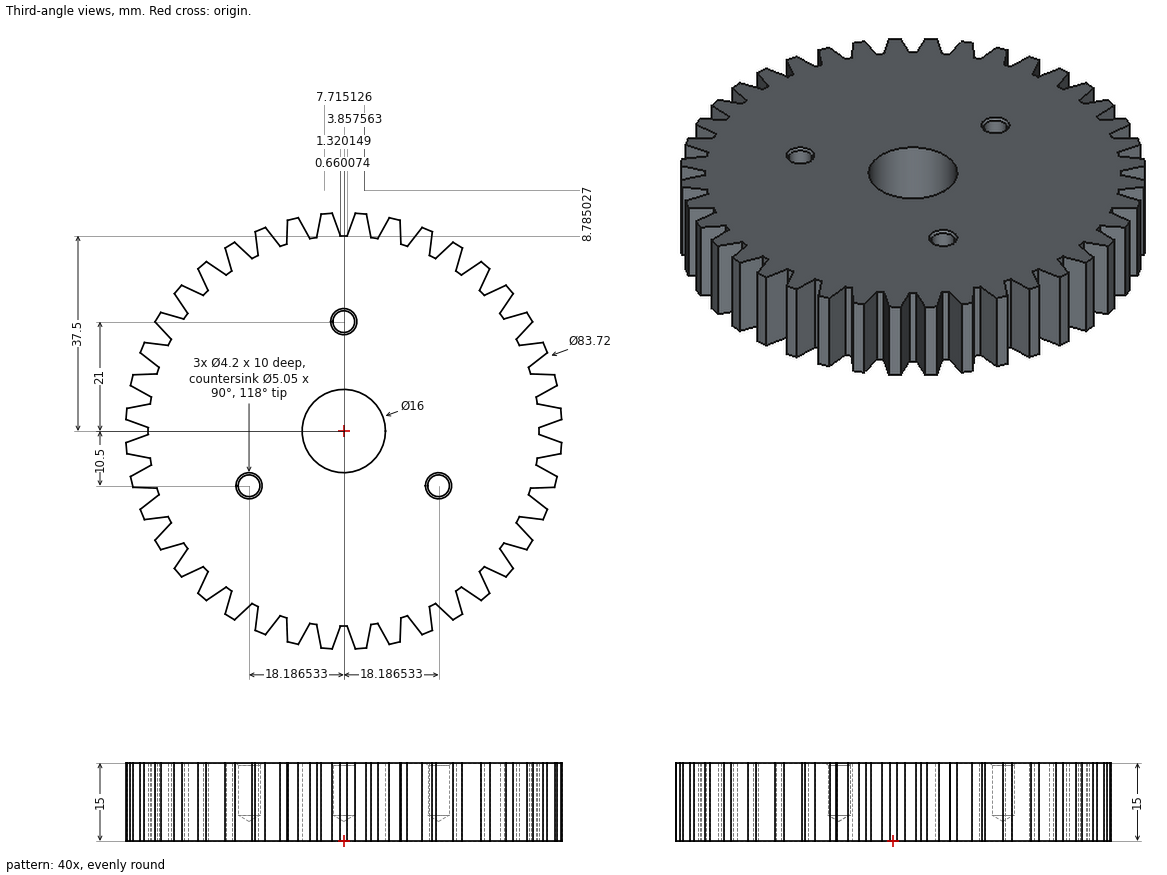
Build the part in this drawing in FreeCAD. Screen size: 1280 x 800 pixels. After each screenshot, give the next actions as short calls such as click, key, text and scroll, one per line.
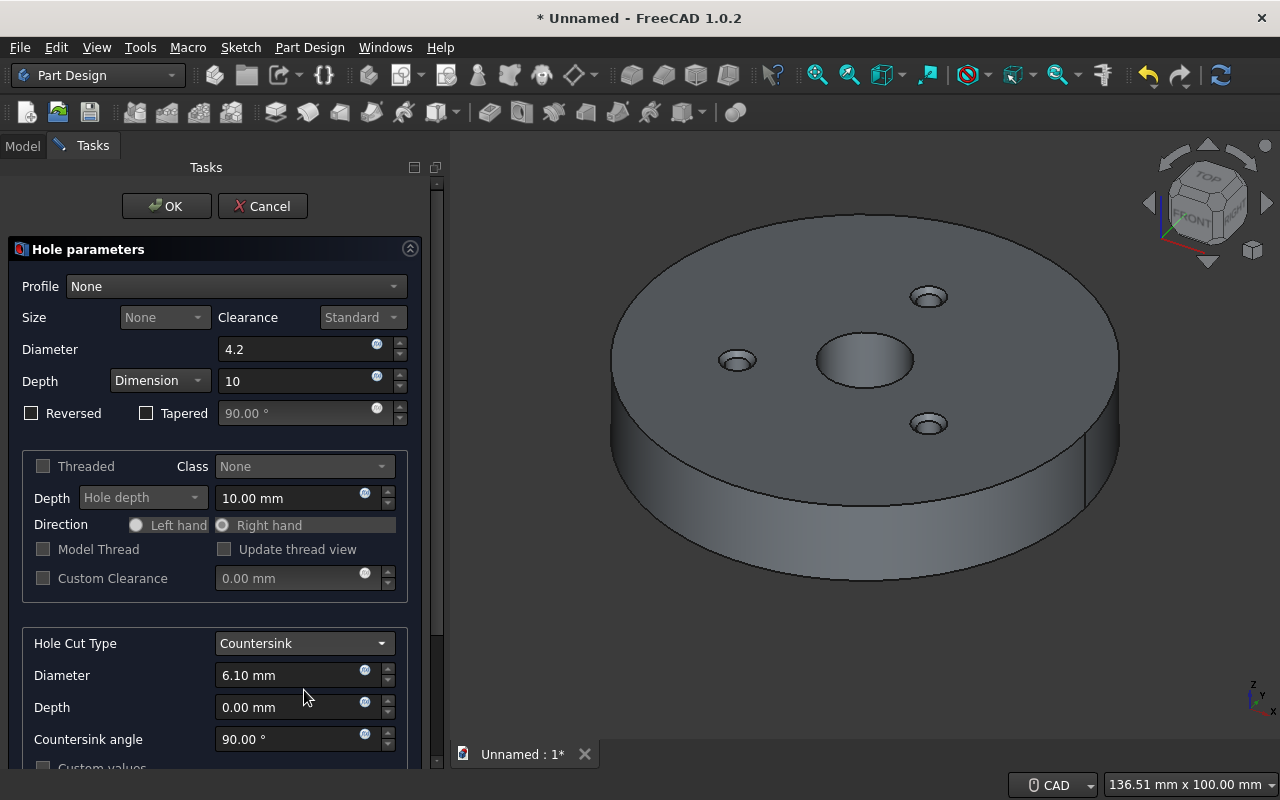
triple_click(298, 675)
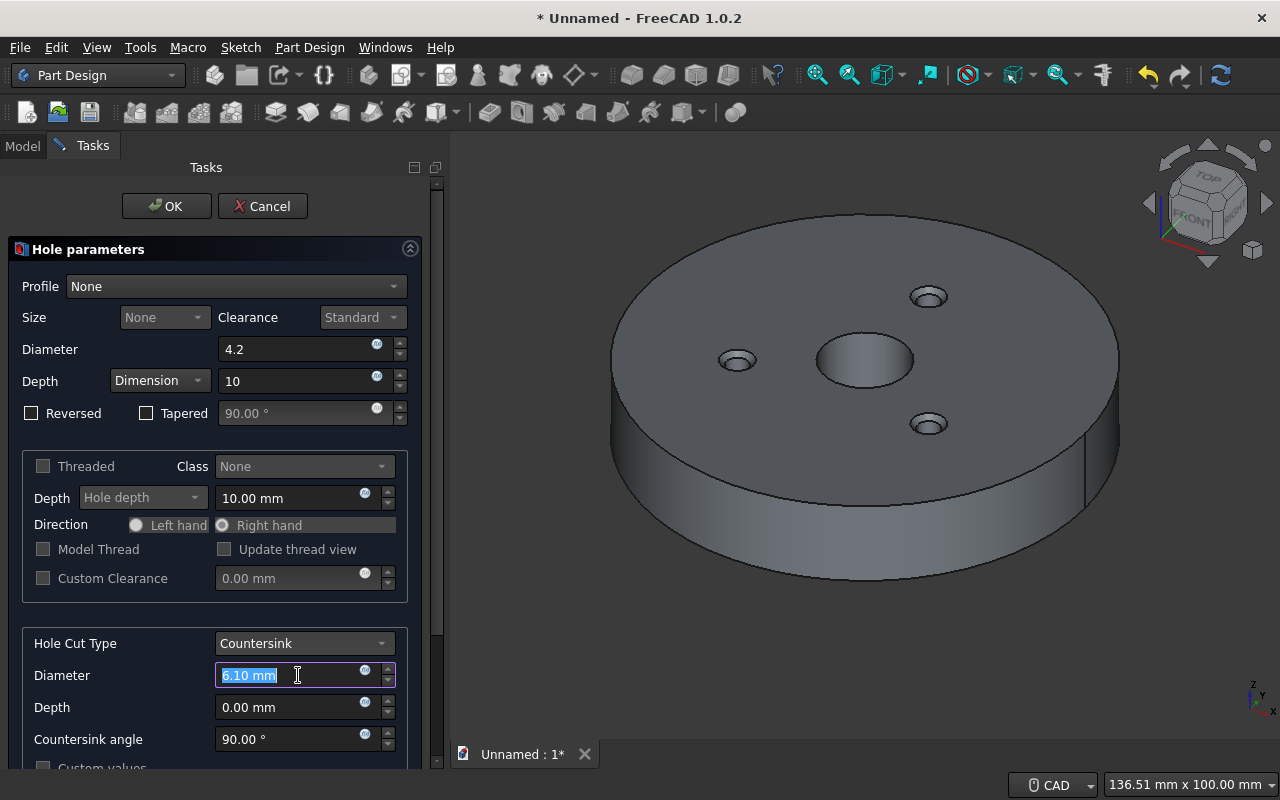
text(5.05)
key(Tab)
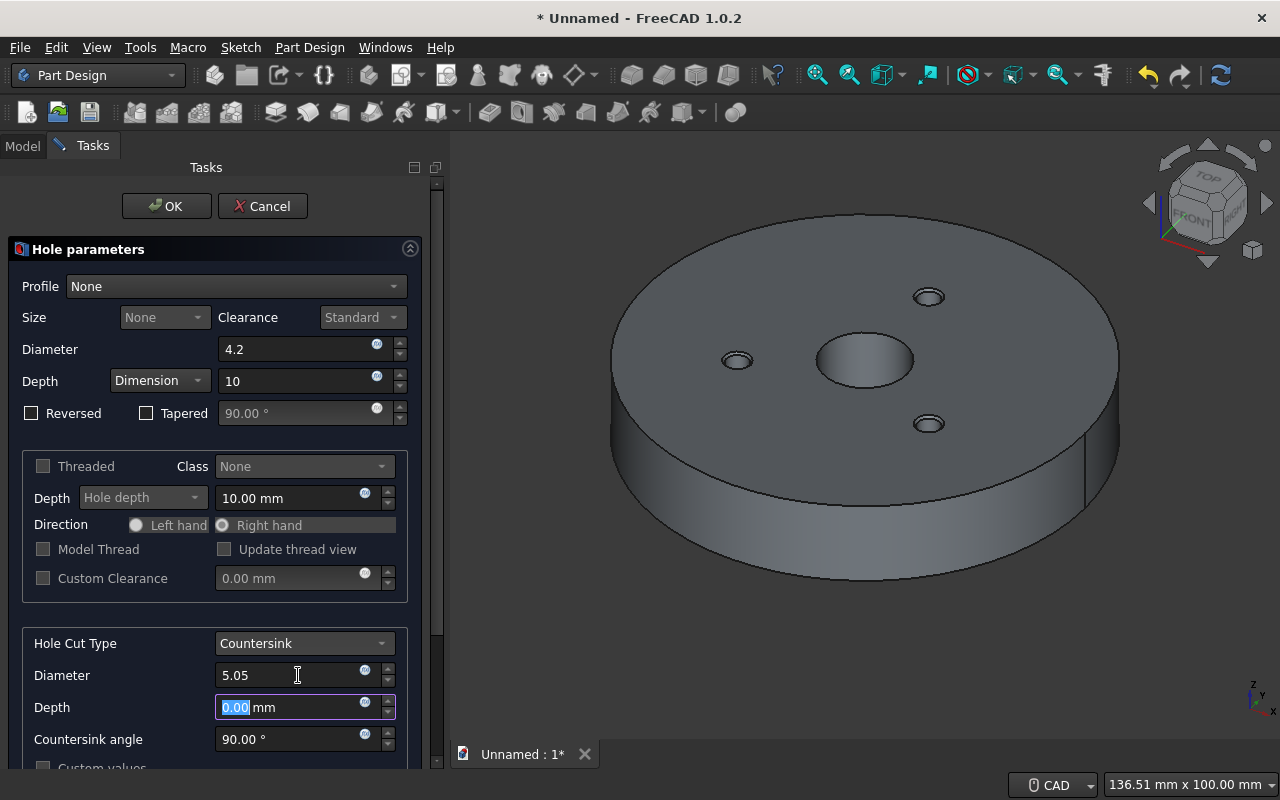
click(167, 206)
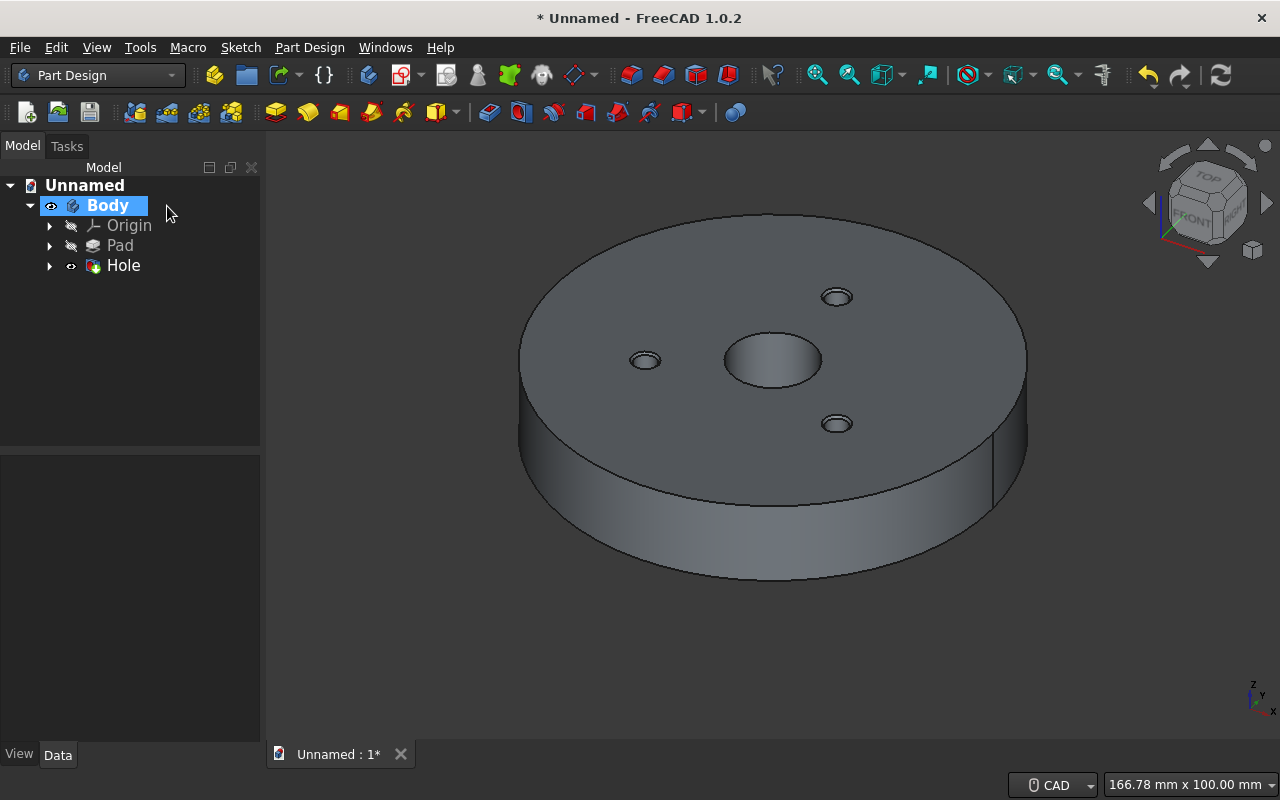
click(402, 76)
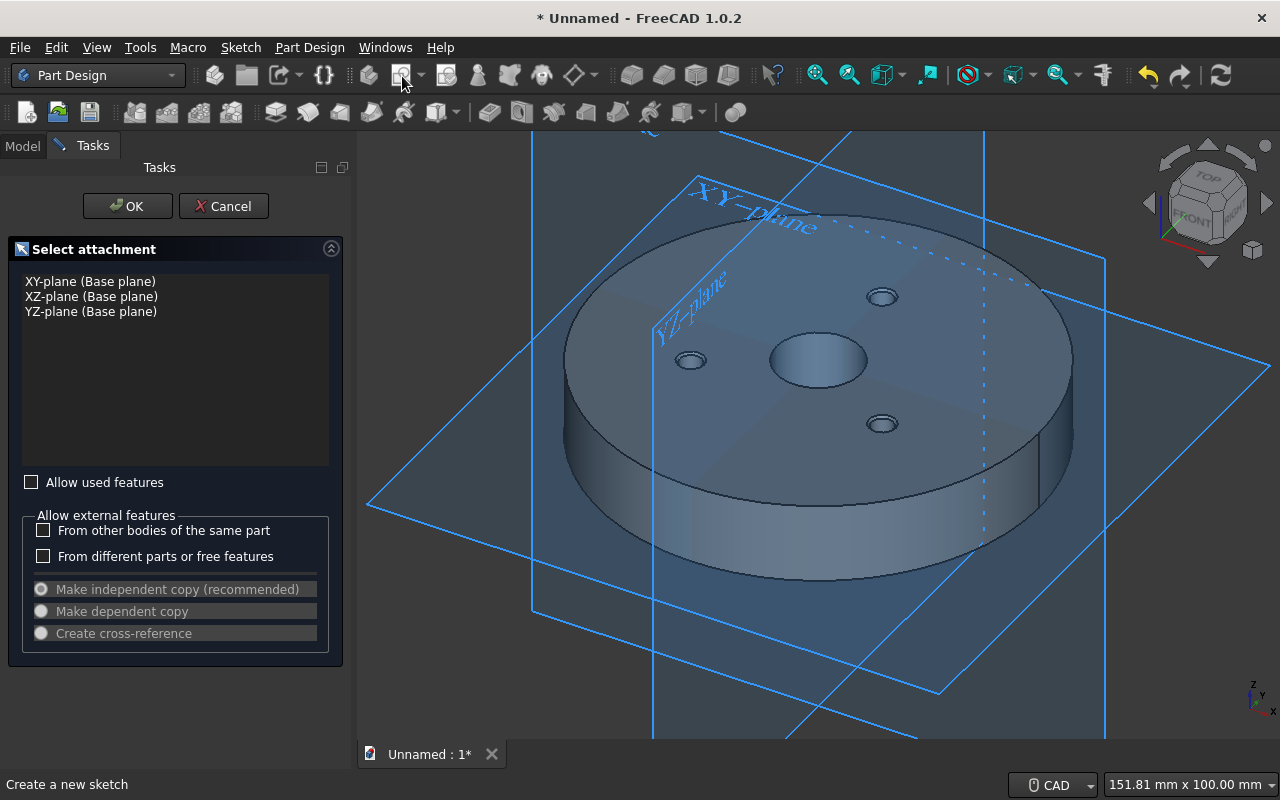
click(82, 282)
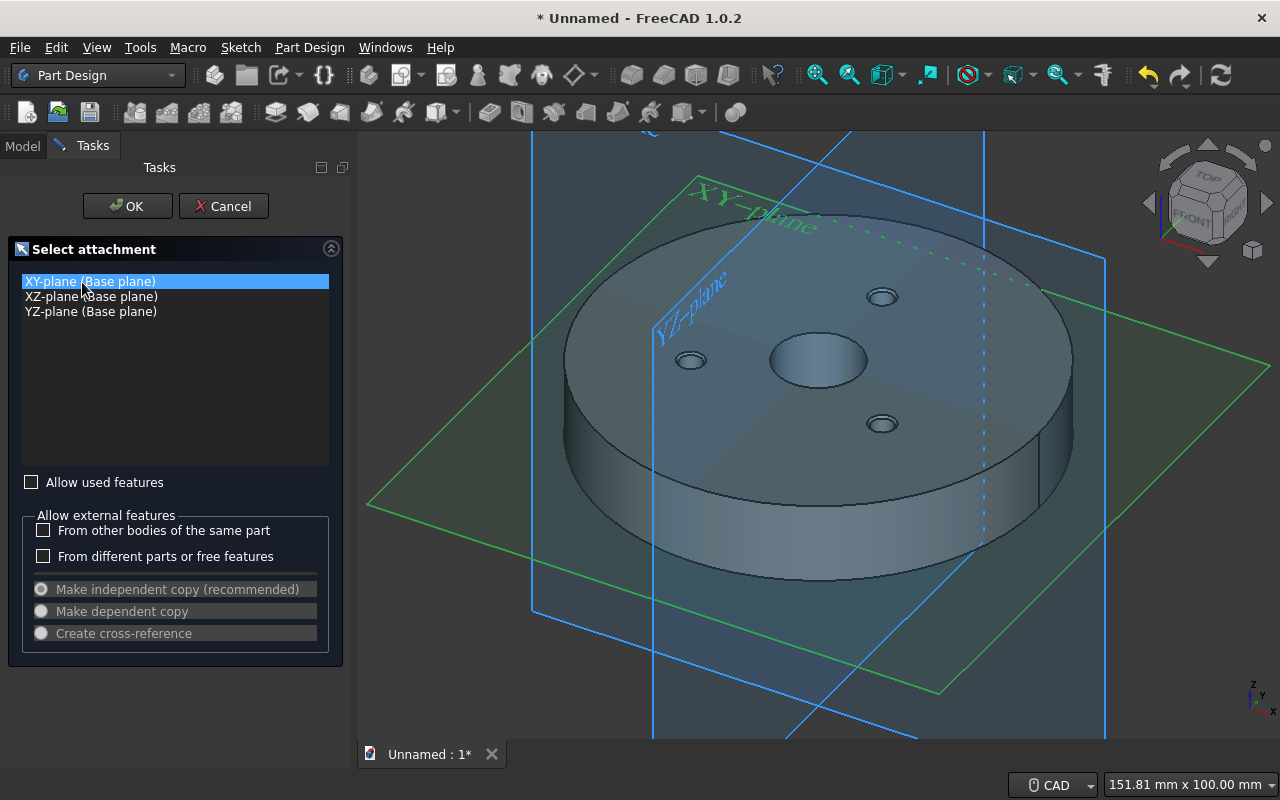
click(128, 206)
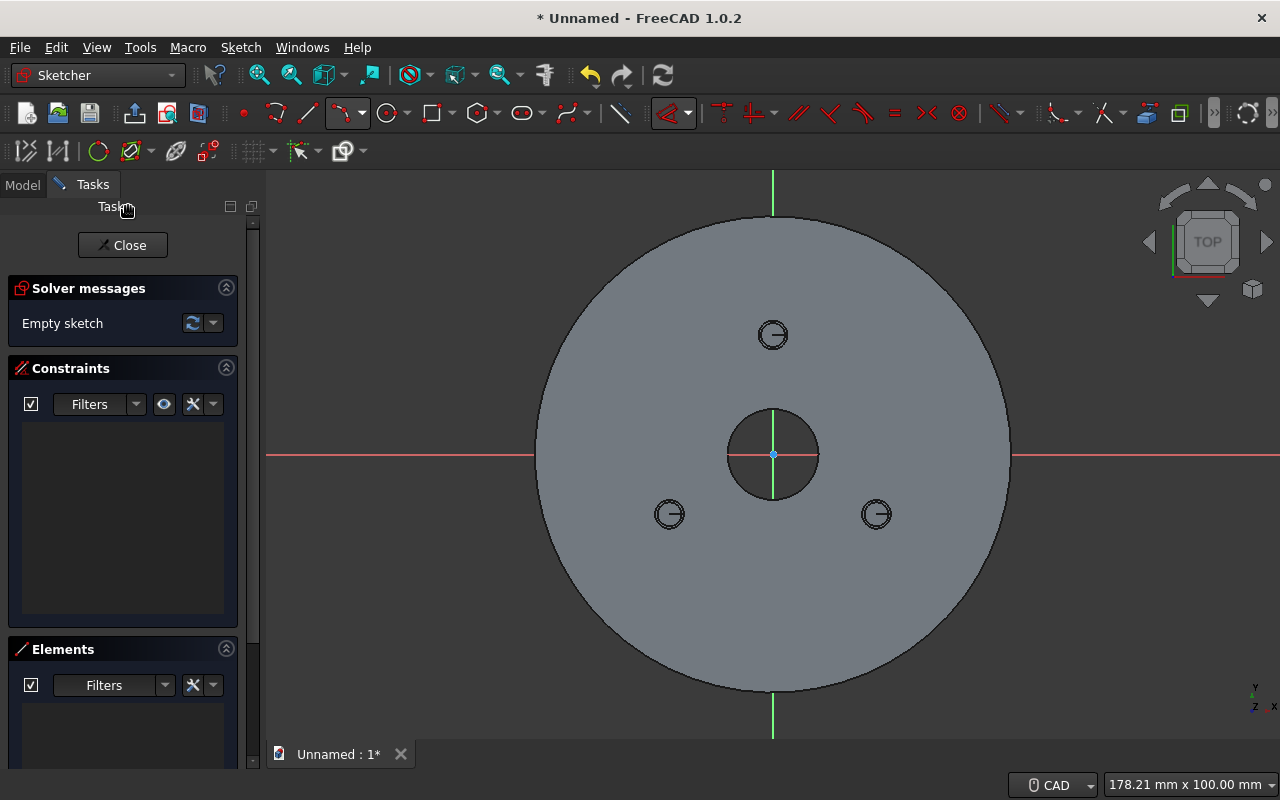
click(200, 114)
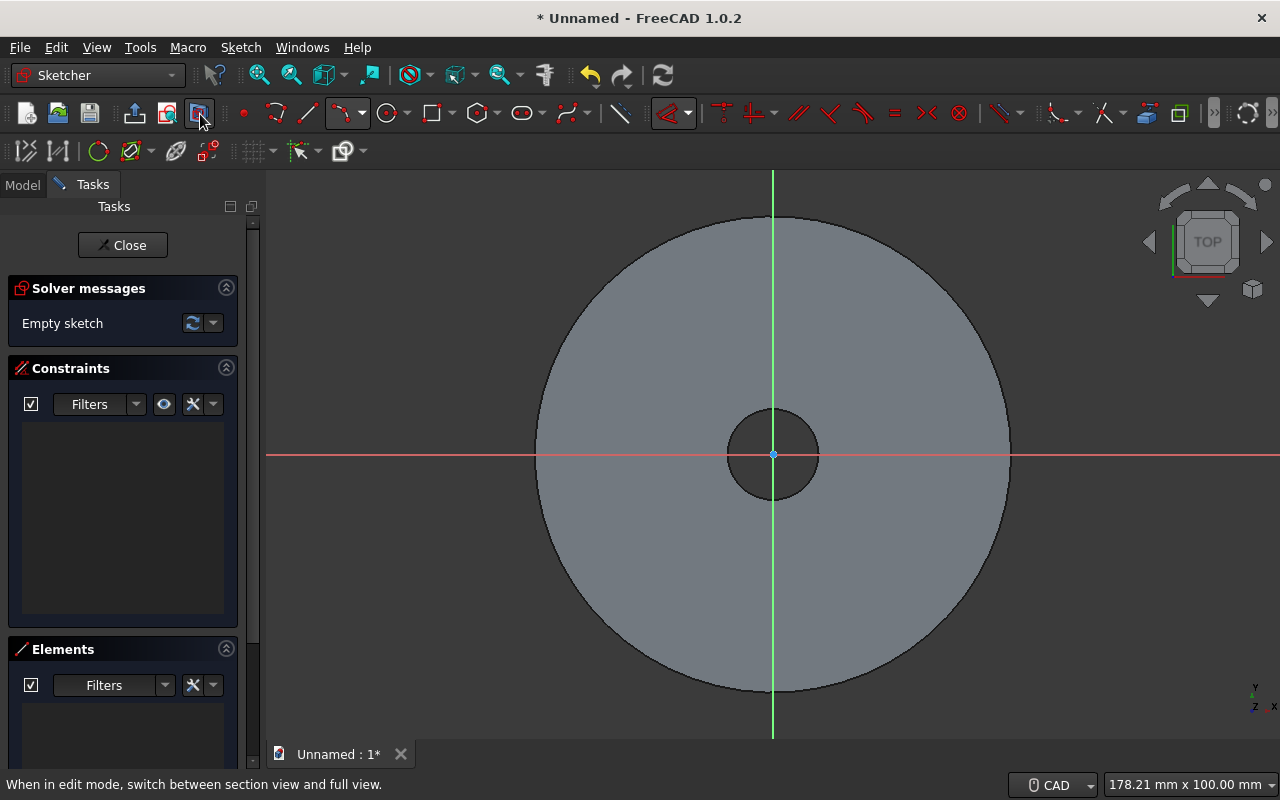
scroll(704, 454, down, 5)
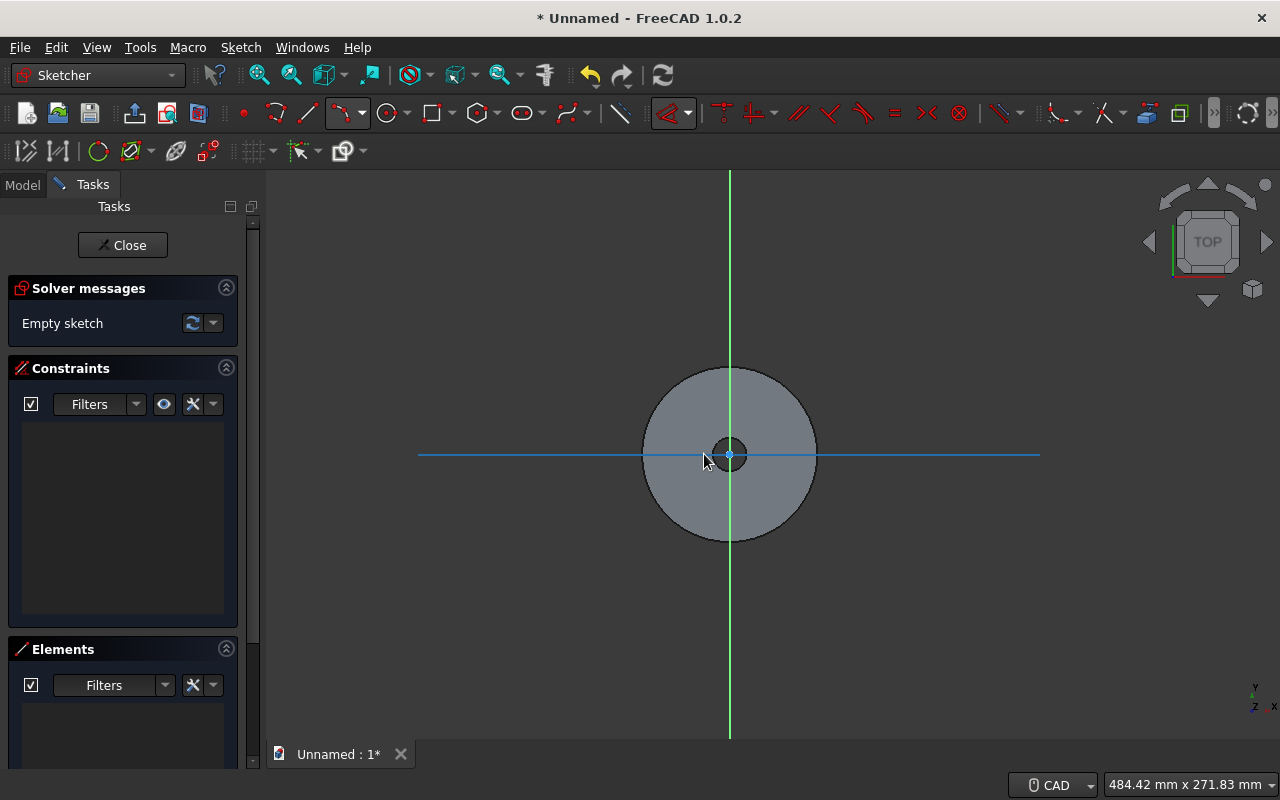
scroll(731, 362, up, 15)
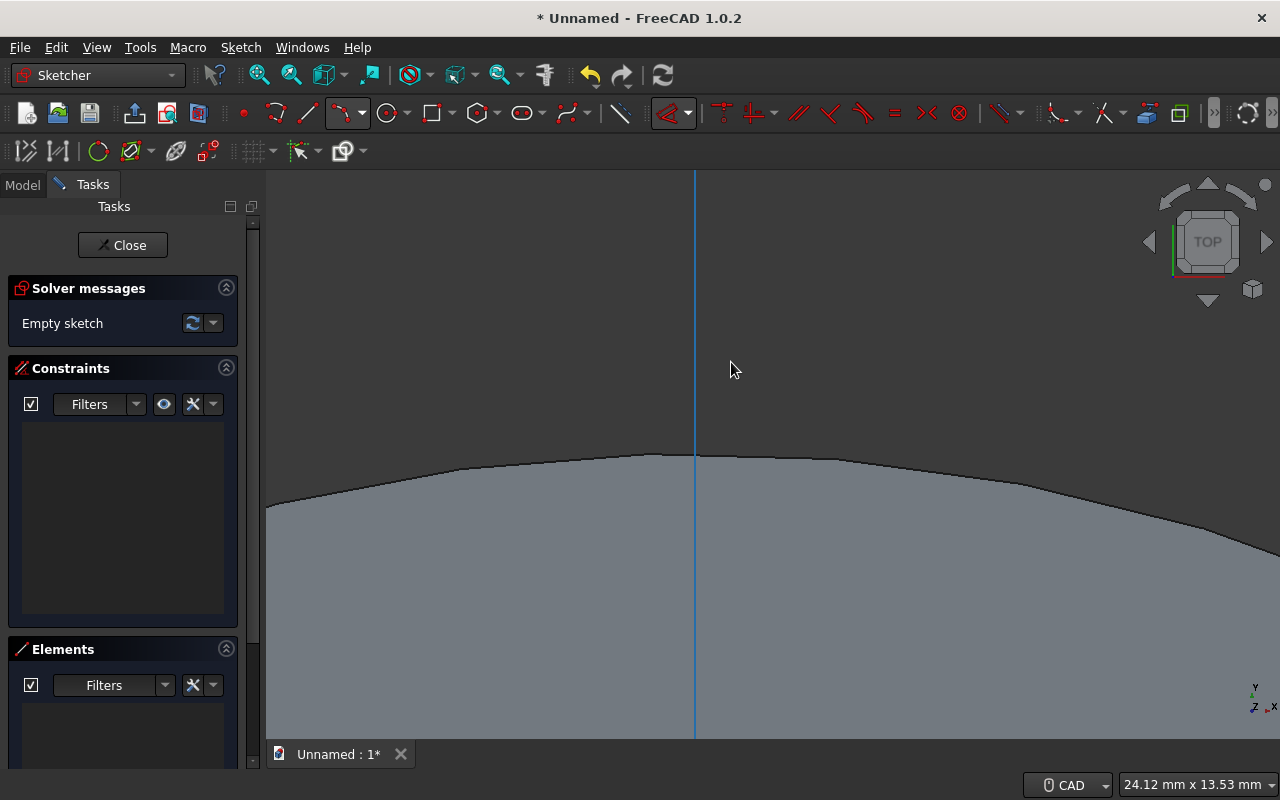
key(g)
key(m)